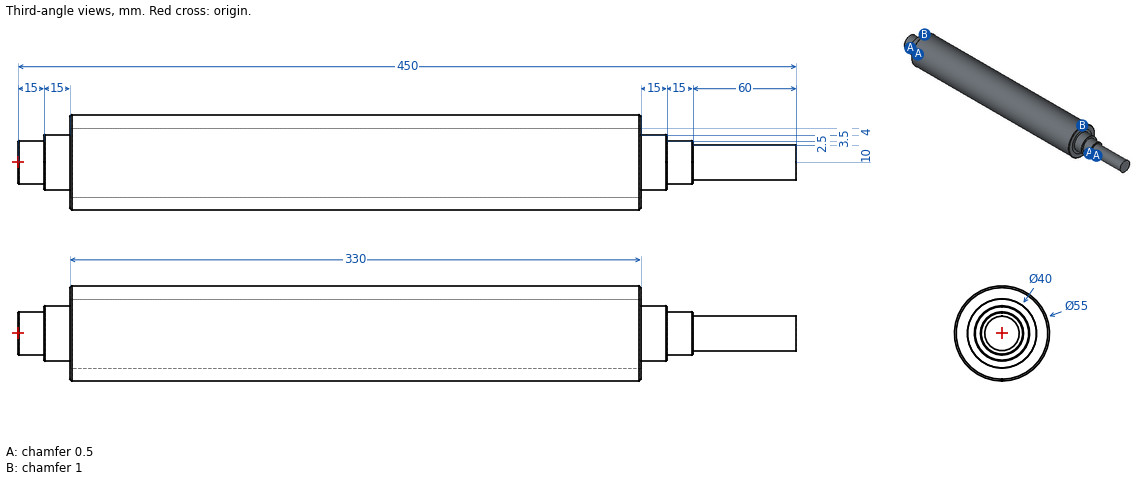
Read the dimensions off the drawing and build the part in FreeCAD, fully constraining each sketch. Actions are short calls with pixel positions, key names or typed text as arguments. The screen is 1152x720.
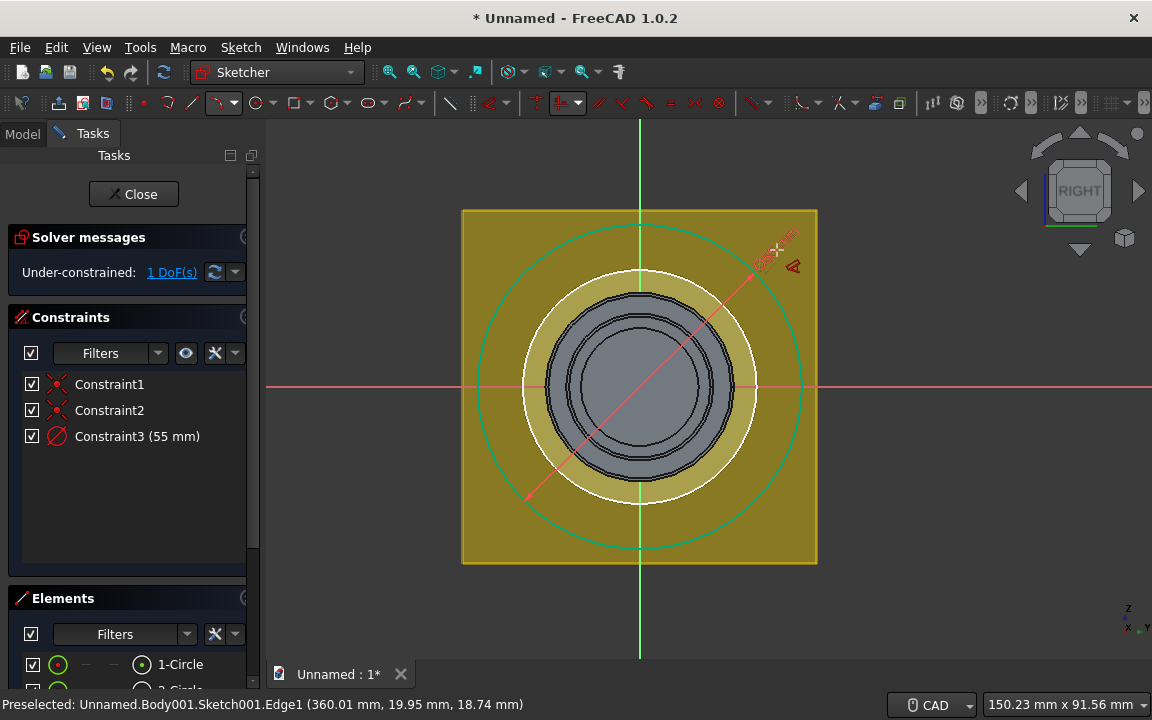
click(722, 304)
click(745, 281)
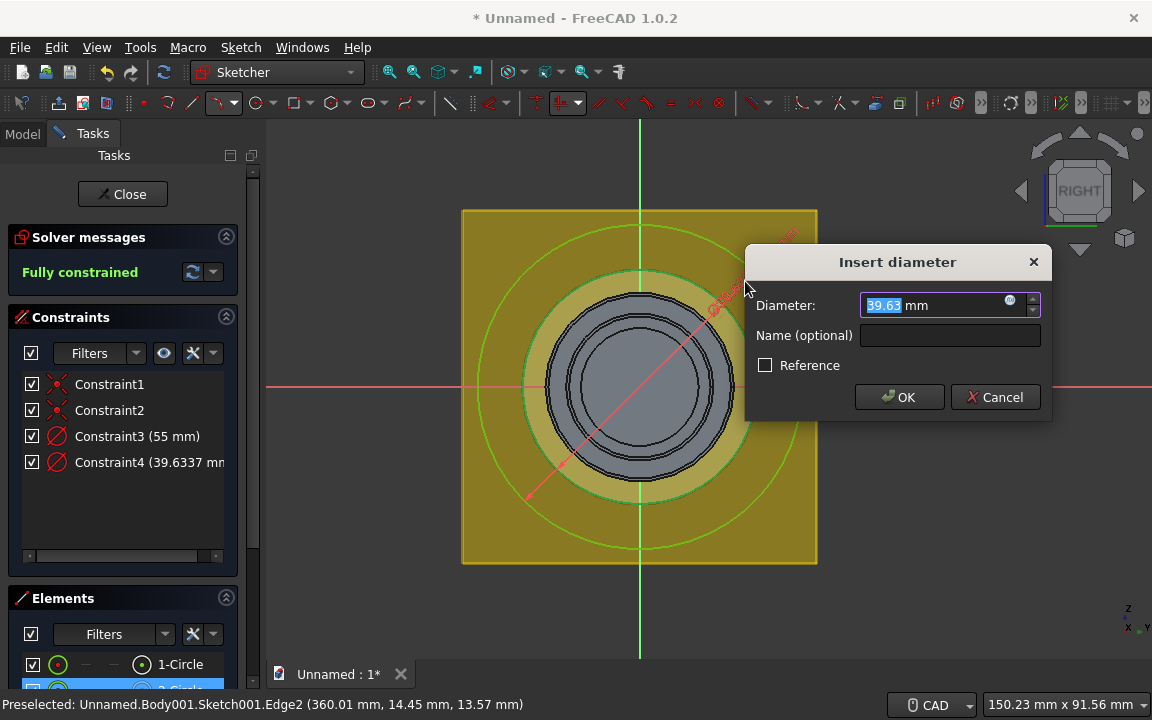
text(40)
key(Return)
key(Escape)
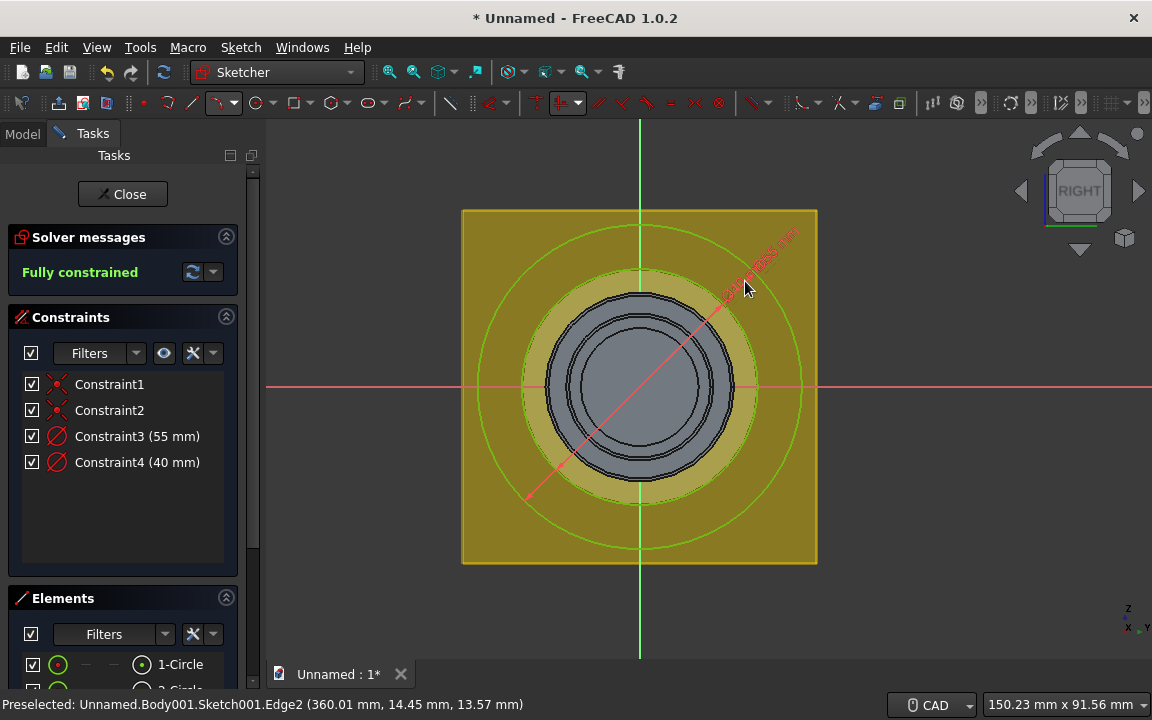
click(123, 194)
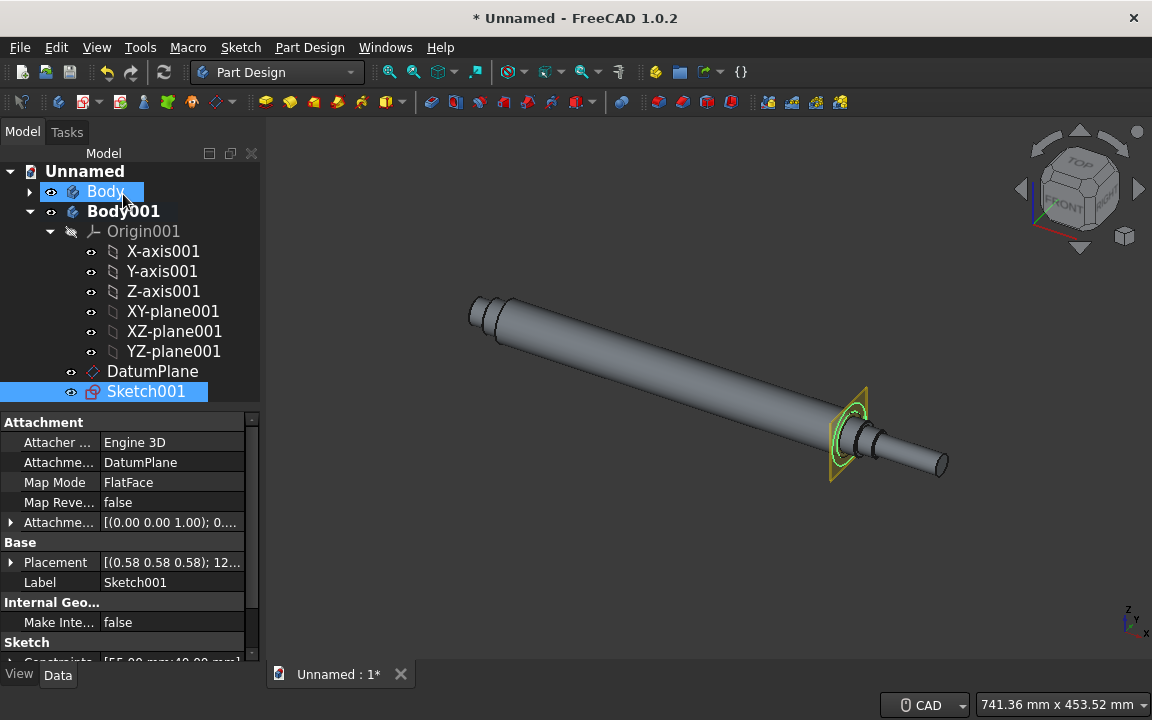
click(266, 102)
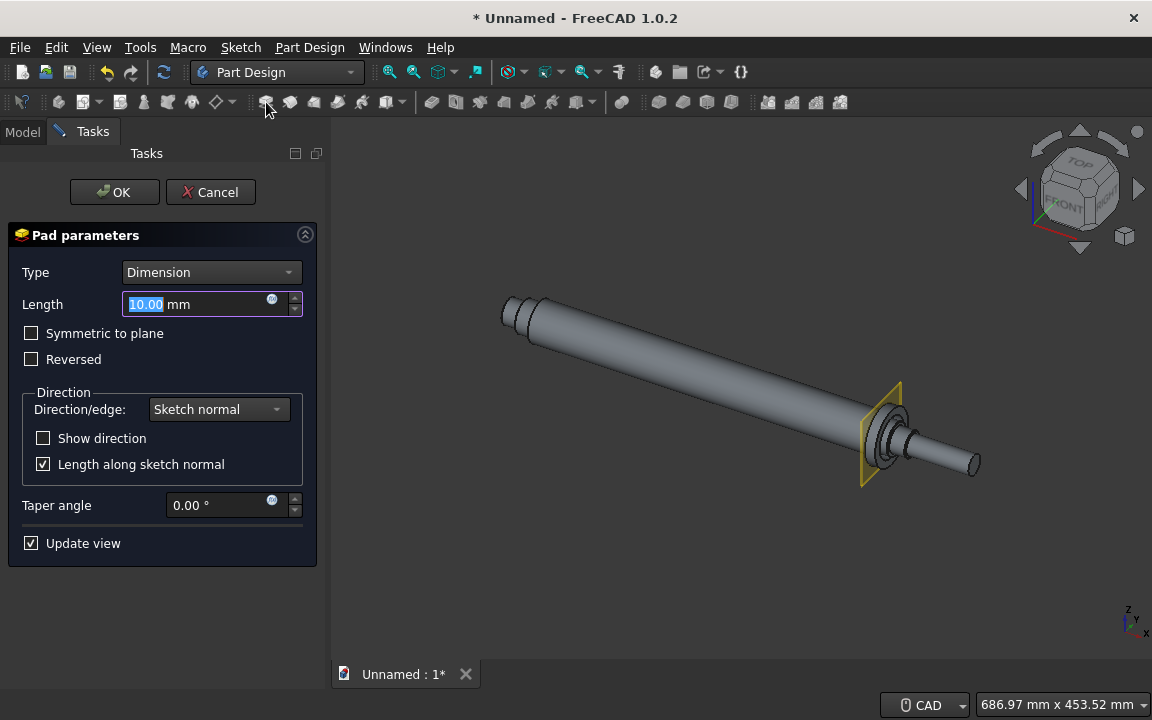
text(330)
key(Tab)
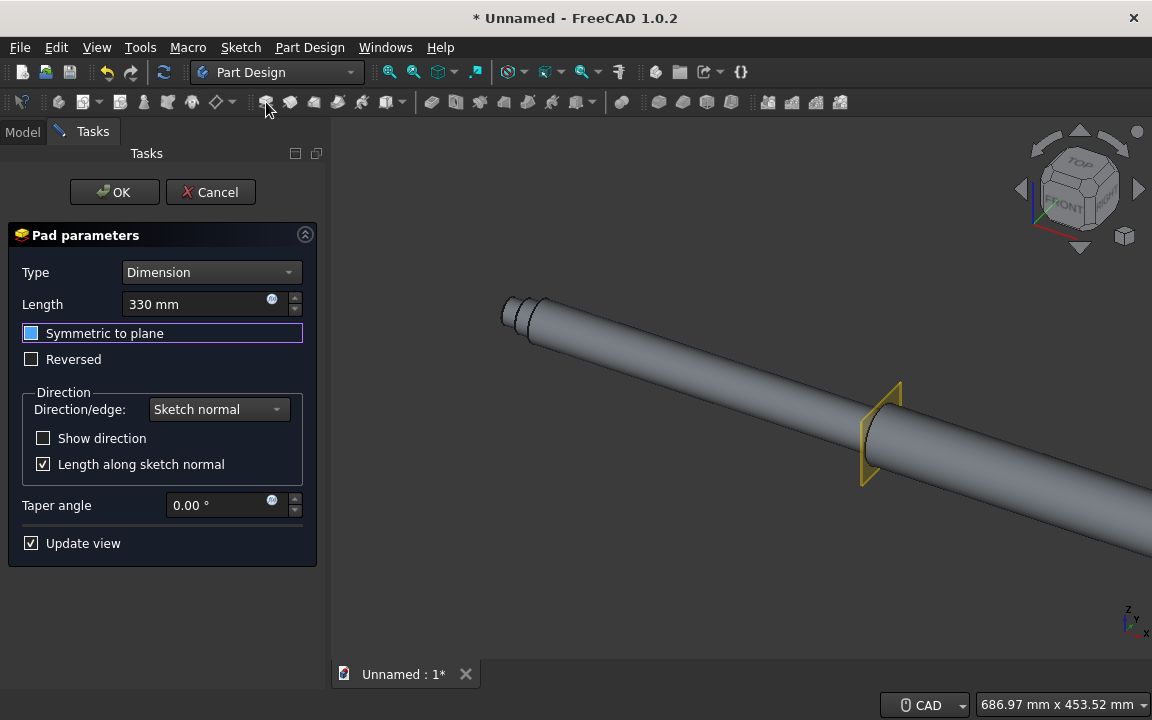
click(30, 359)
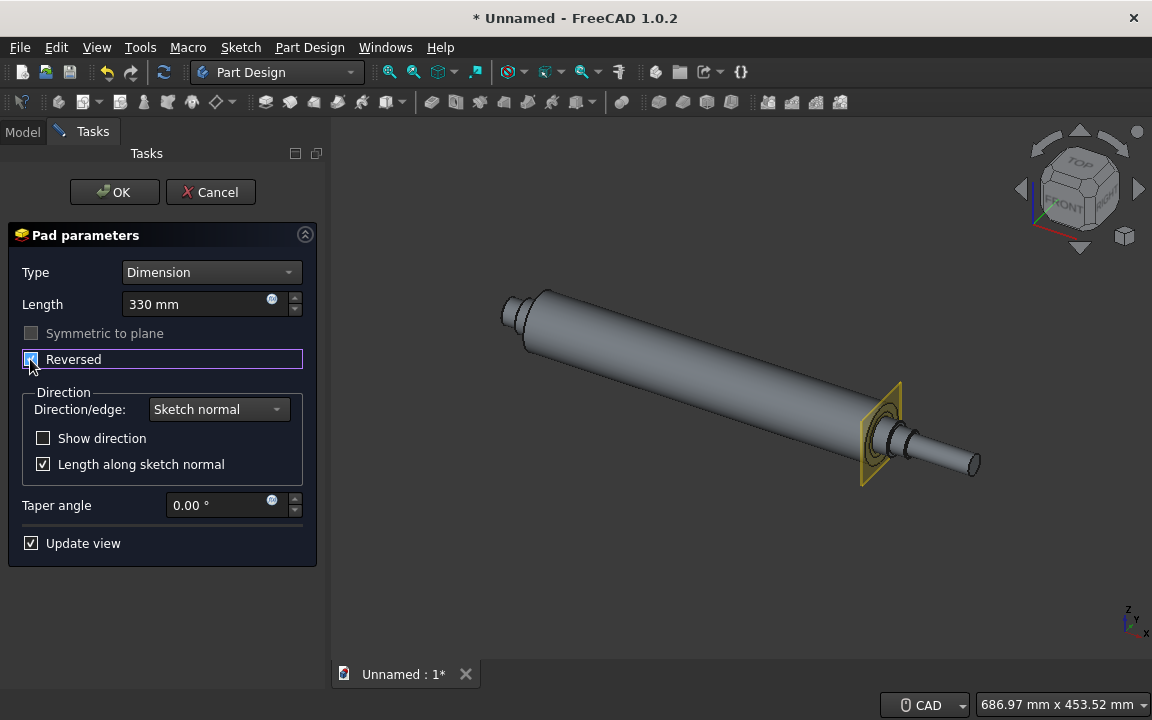
click(115, 192)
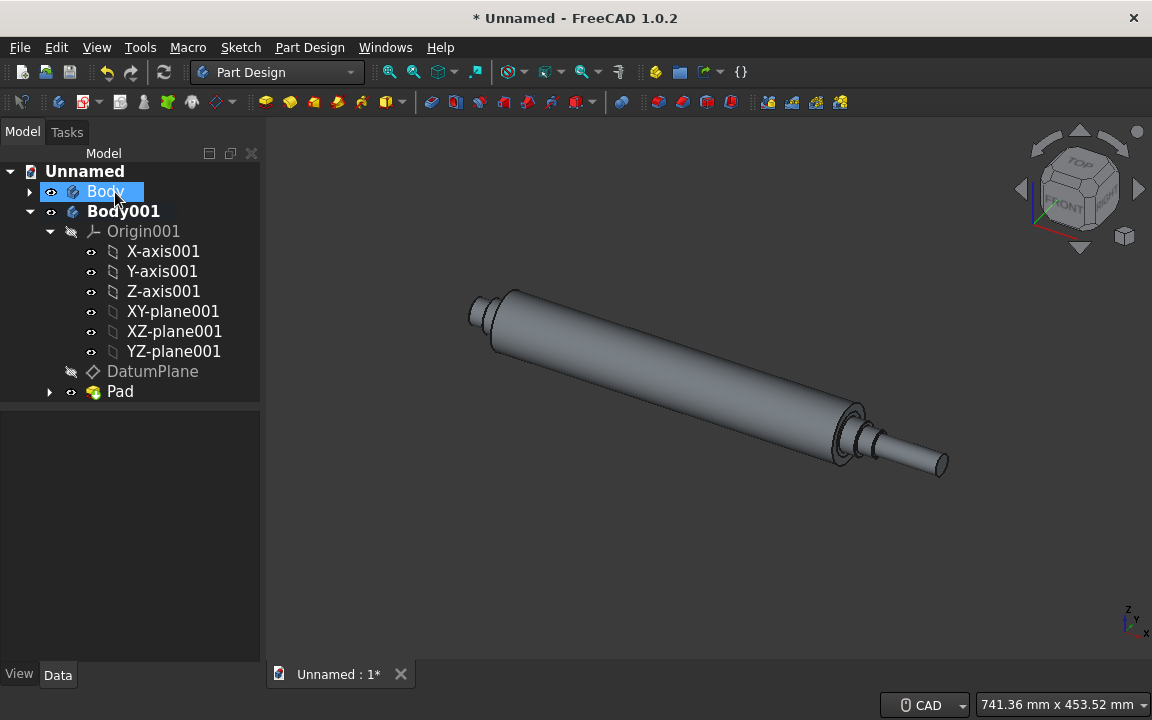
click(390, 72)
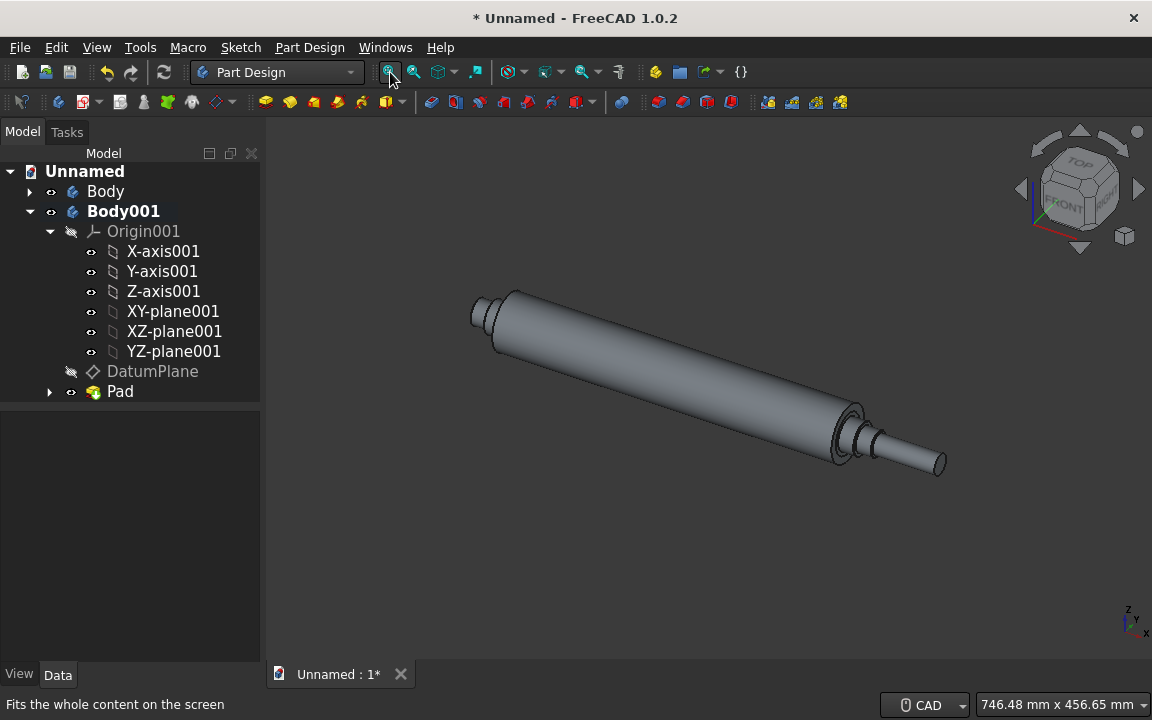
click(831, 449)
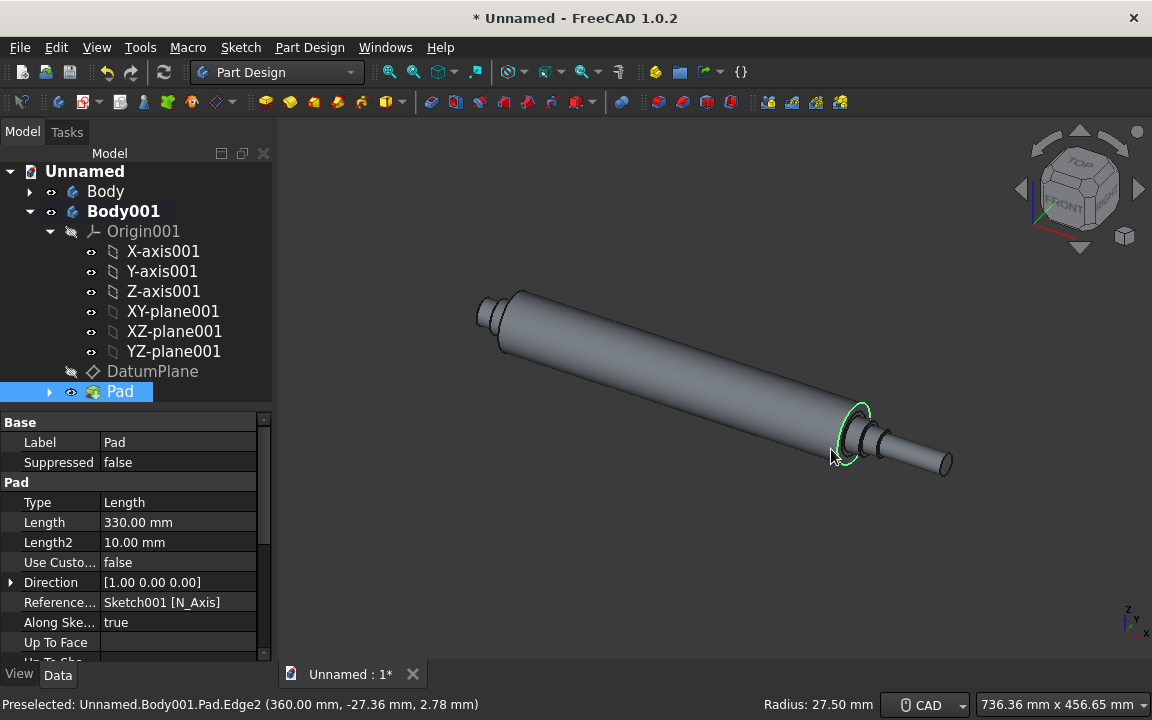
click(498, 337, ctrl)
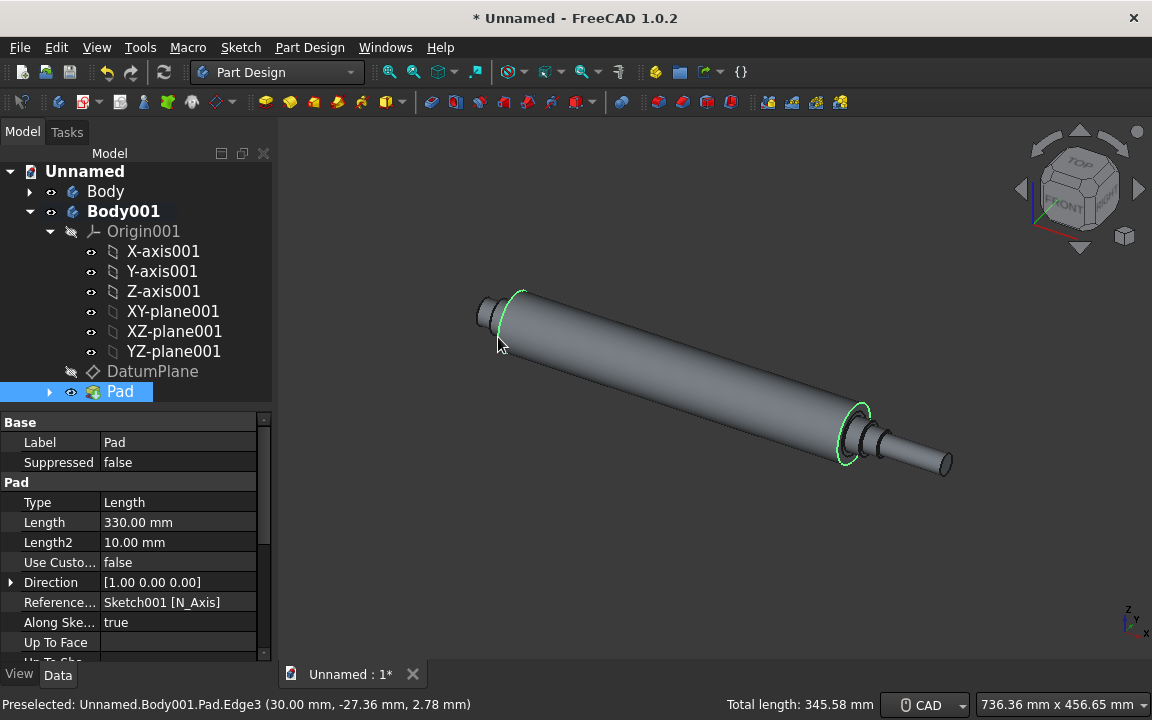
click(684, 102)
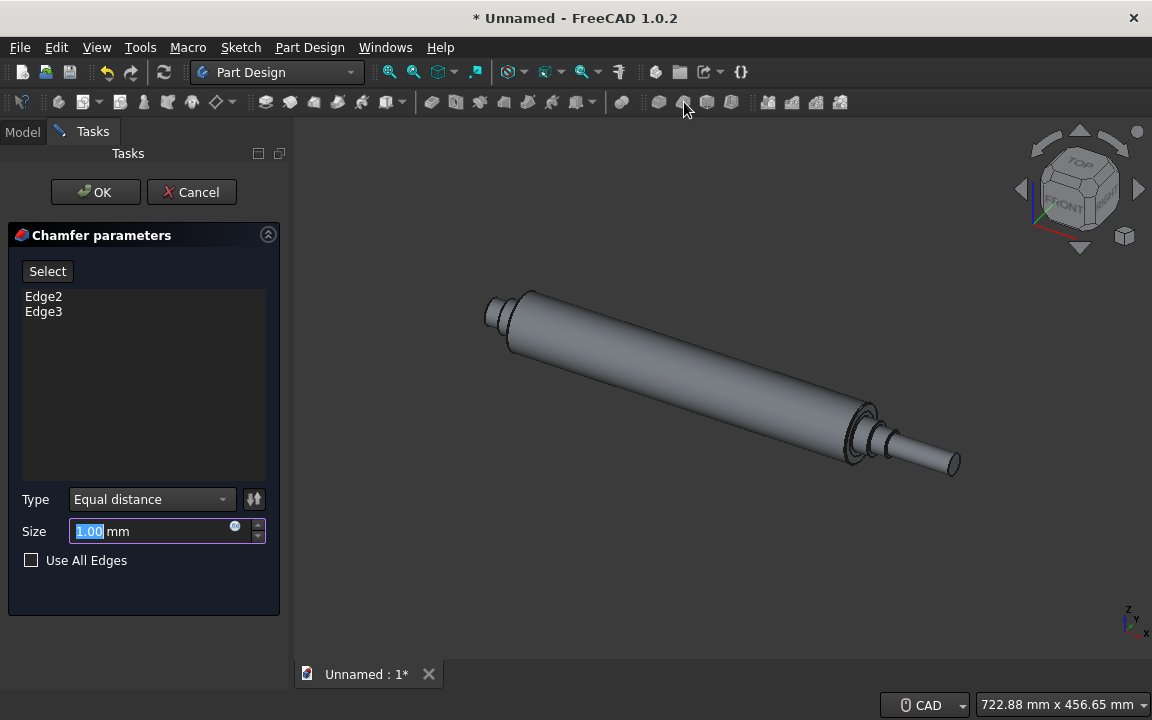
text(1)
key(Tab)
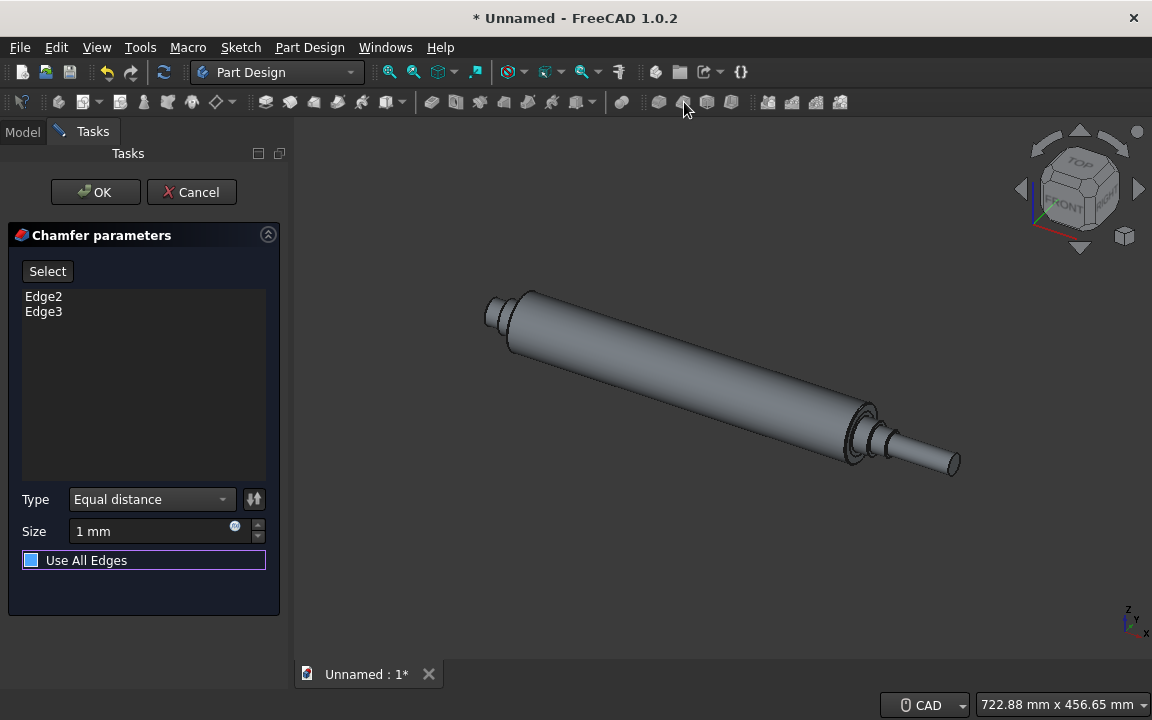
click(96, 192)